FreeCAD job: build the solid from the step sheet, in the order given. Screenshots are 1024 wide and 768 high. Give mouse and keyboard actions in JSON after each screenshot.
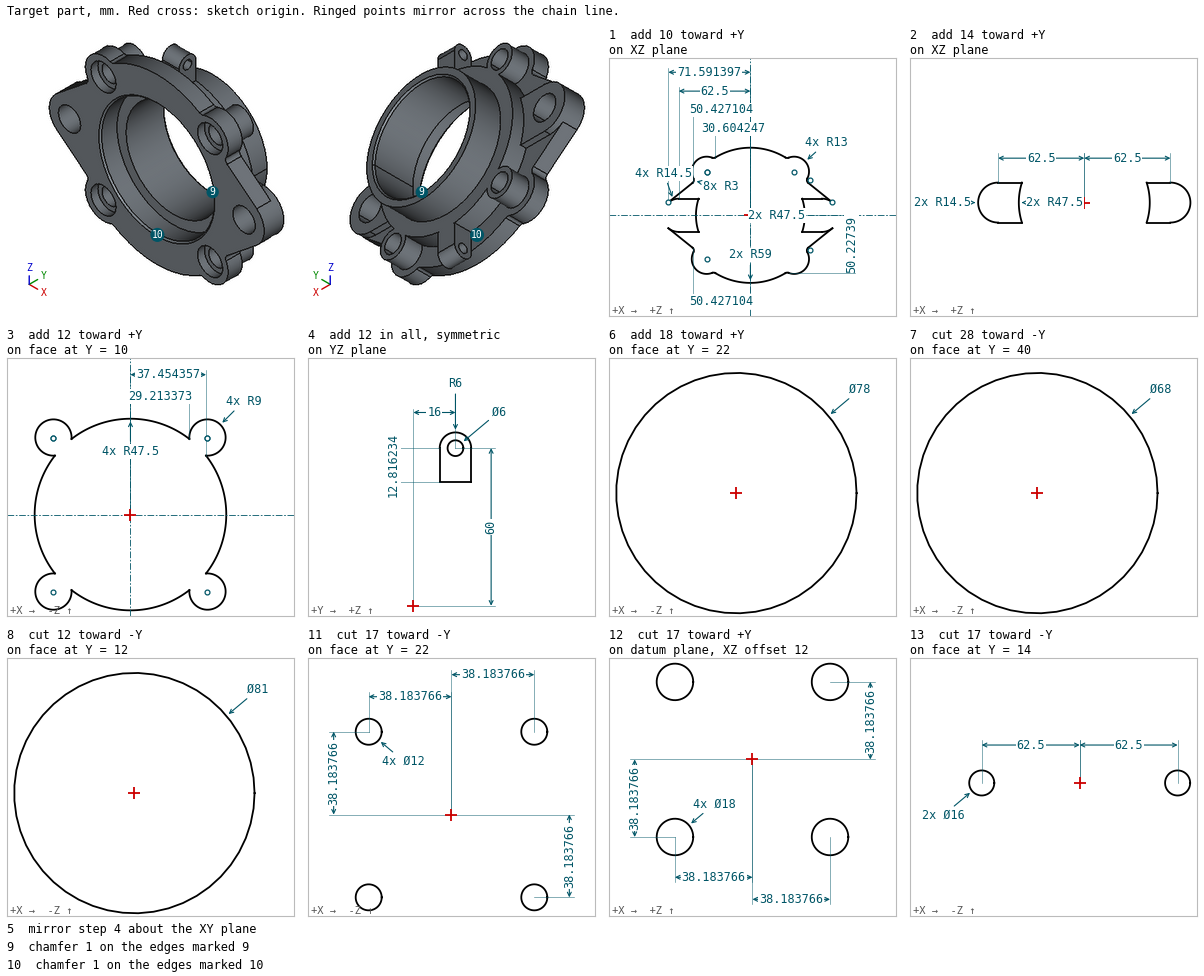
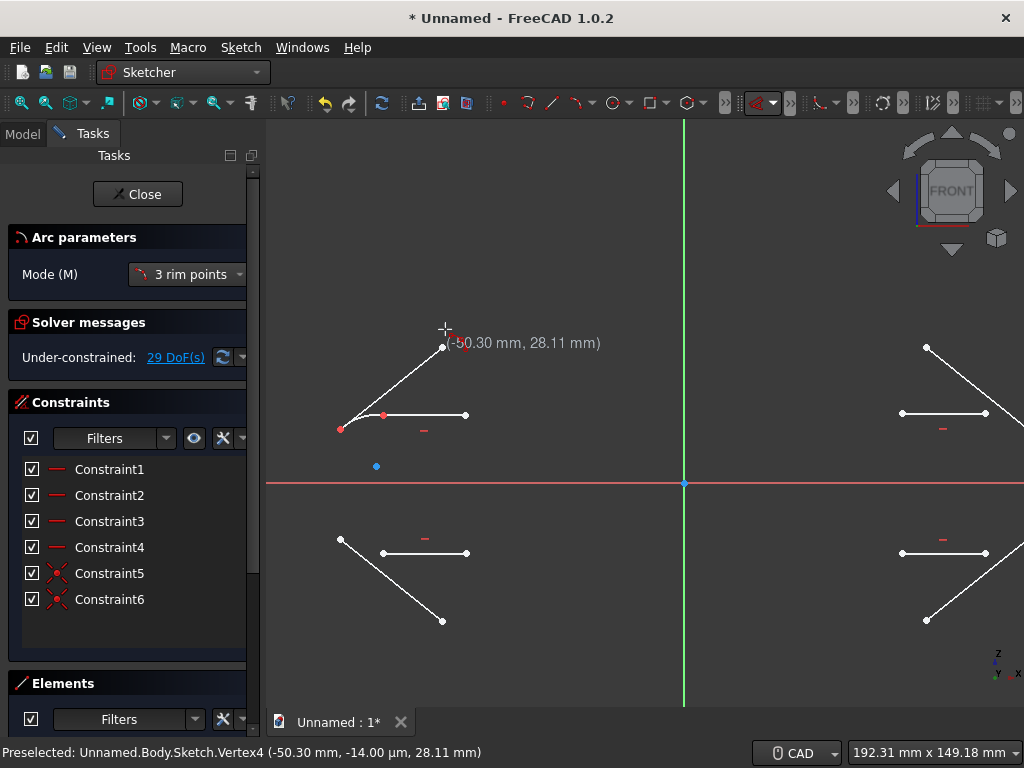
{"action": "left_click", "coordinate": [445, 329]}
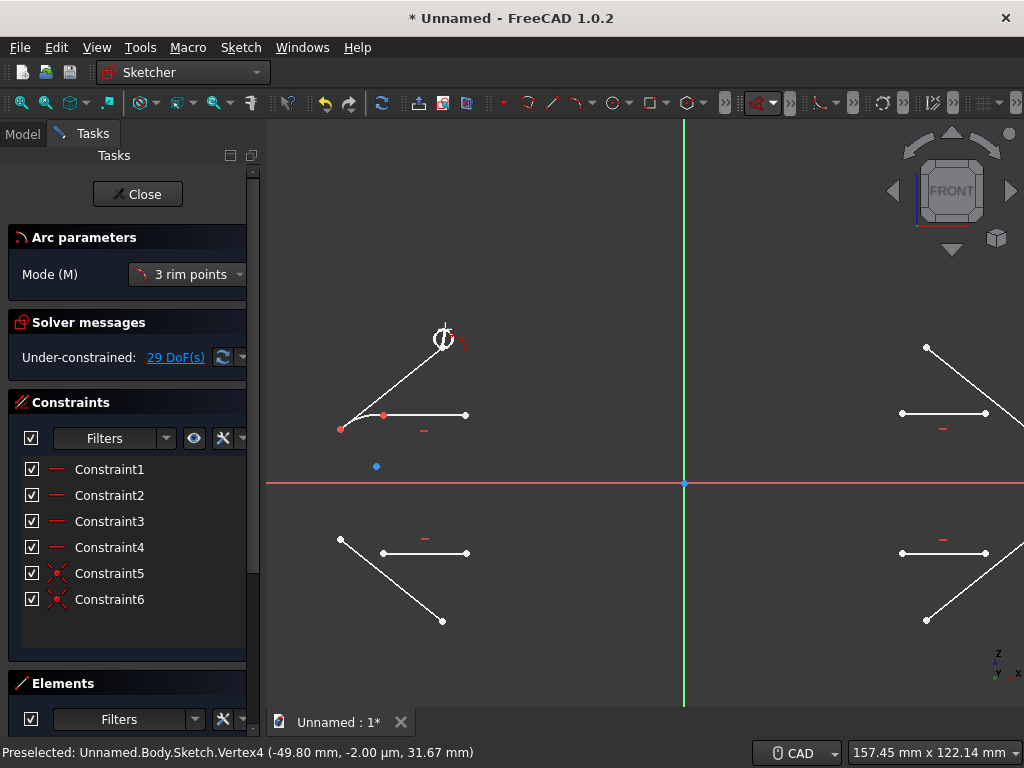
{"action": "scroll", "coordinate": [447, 339], "scroll_direction": "up", "scroll_amount": 8}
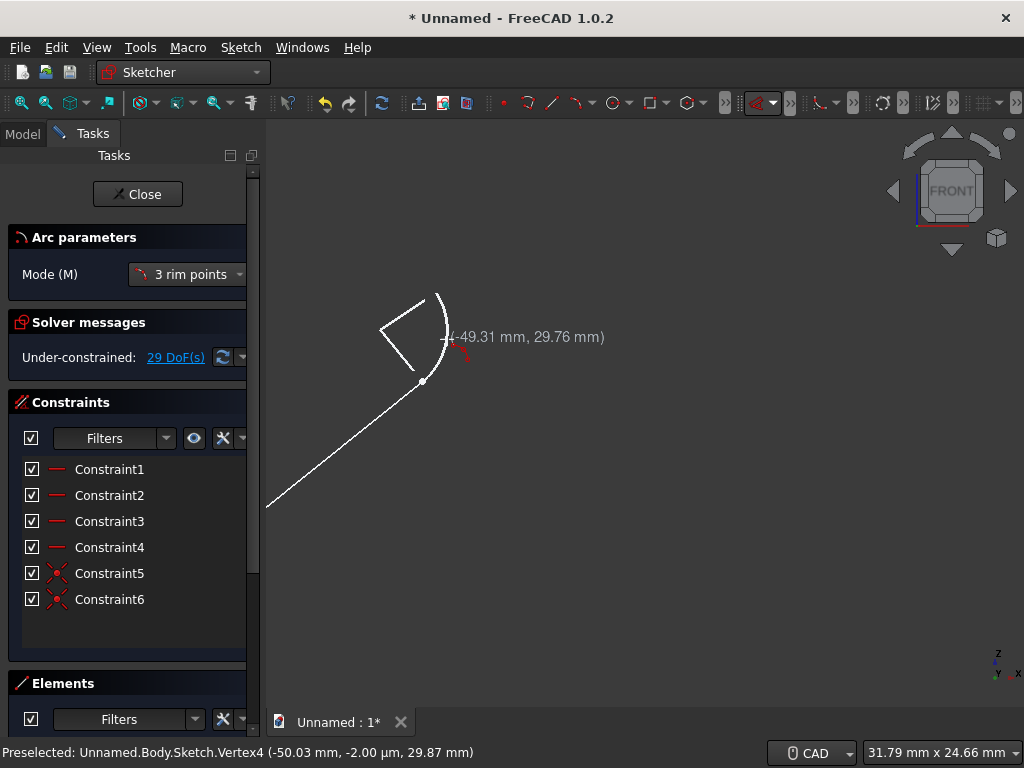
{"action": "left_click", "coordinate": [445, 335]}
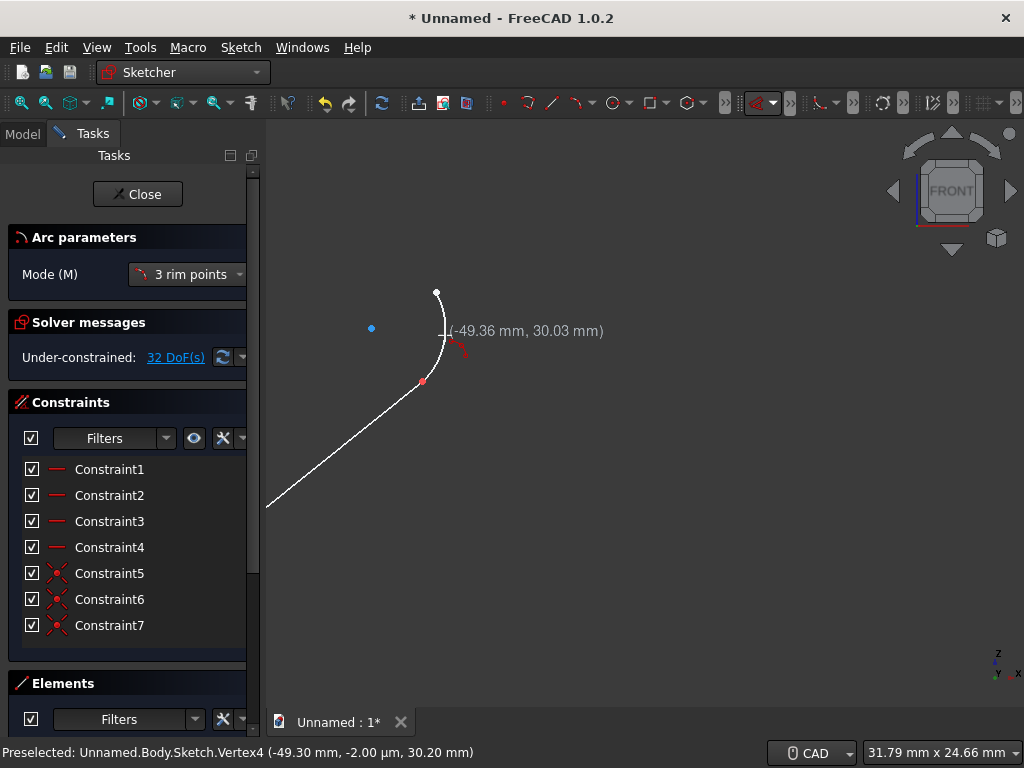
{"action": "scroll", "coordinate": [446, 333], "scroll_direction": "down", "scroll_amount": 11}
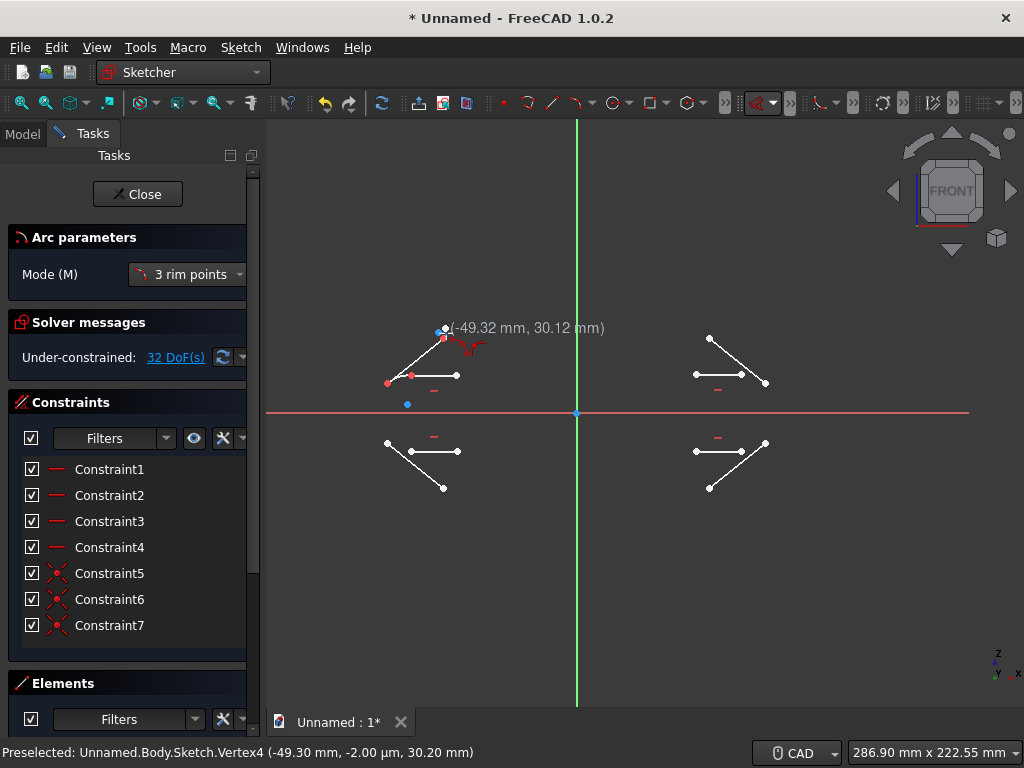
{"action": "scroll", "coordinate": [445, 328], "scroll_direction": "up", "scroll_amount": 4}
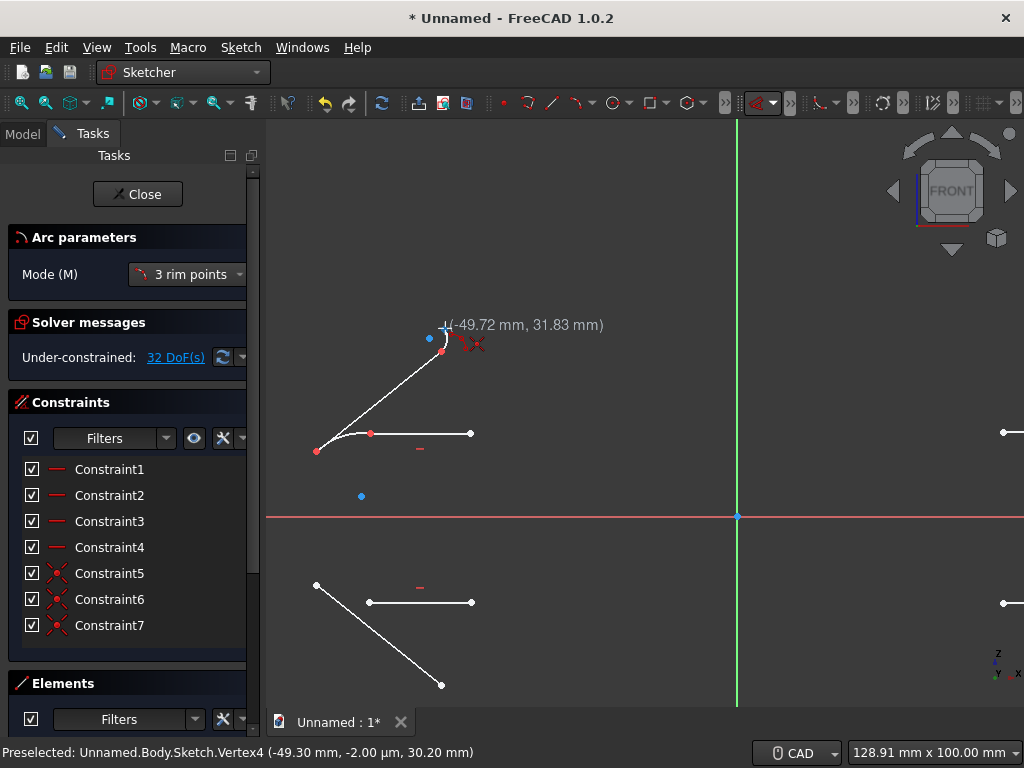
{"action": "left_click", "coordinate": [445, 330]}
{"action": "left_click", "coordinate": [542, 221]}
{"action": "left_click", "coordinate": [456, 241]}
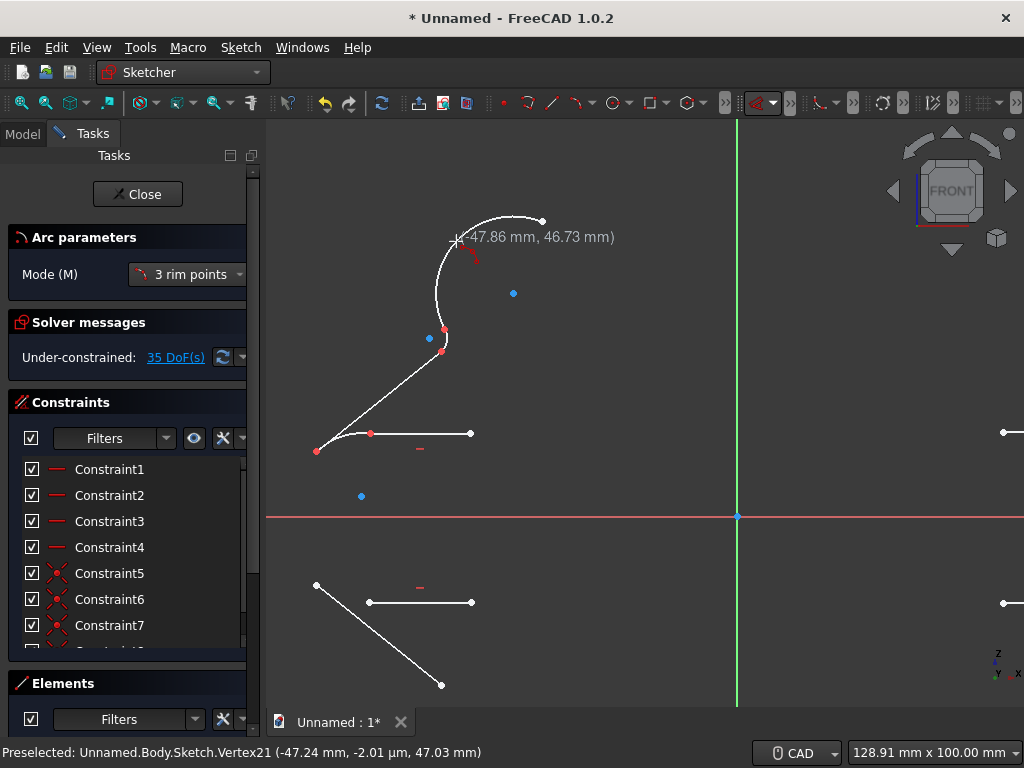
{"action": "left_click", "coordinate": [542, 222]}
{"action": "left_click", "coordinate": [557, 220]}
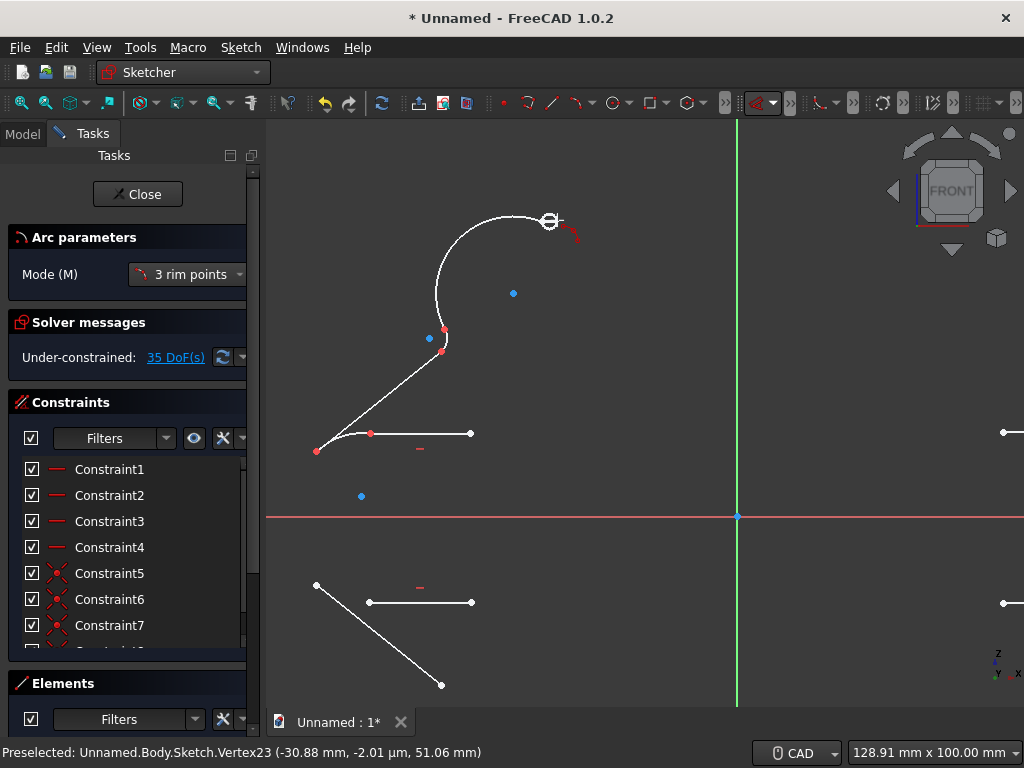
{"action": "scroll", "coordinate": [550, 223], "scroll_direction": "up", "scroll_amount": 11}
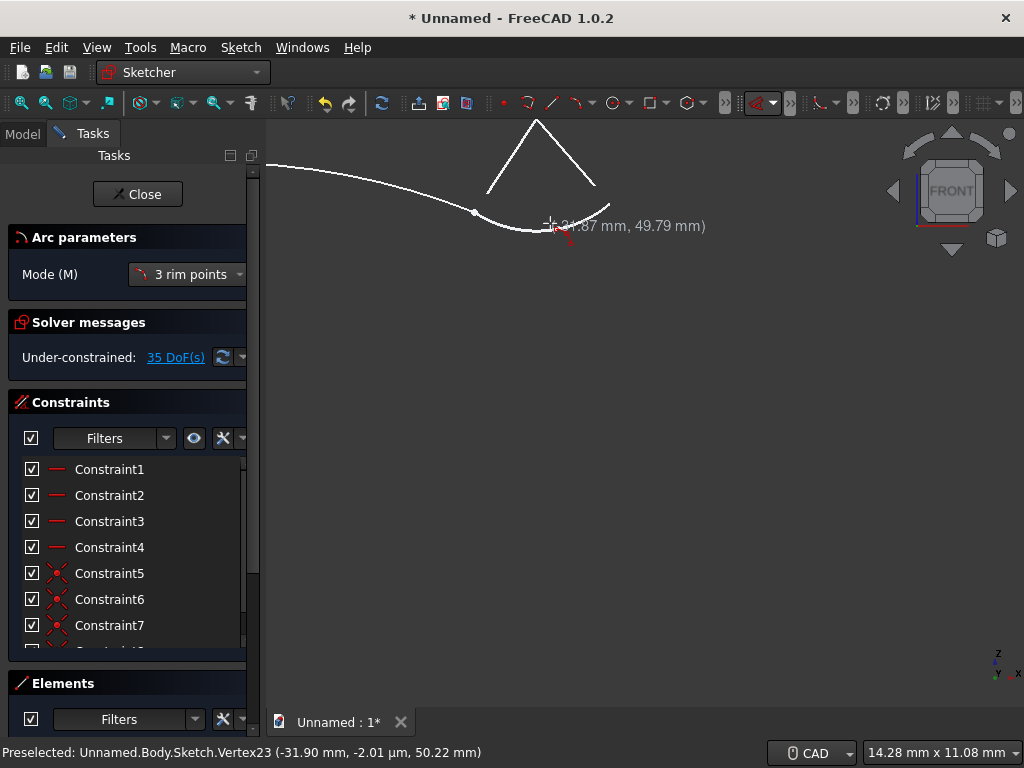
{"action": "left_click", "coordinate": [544, 219]}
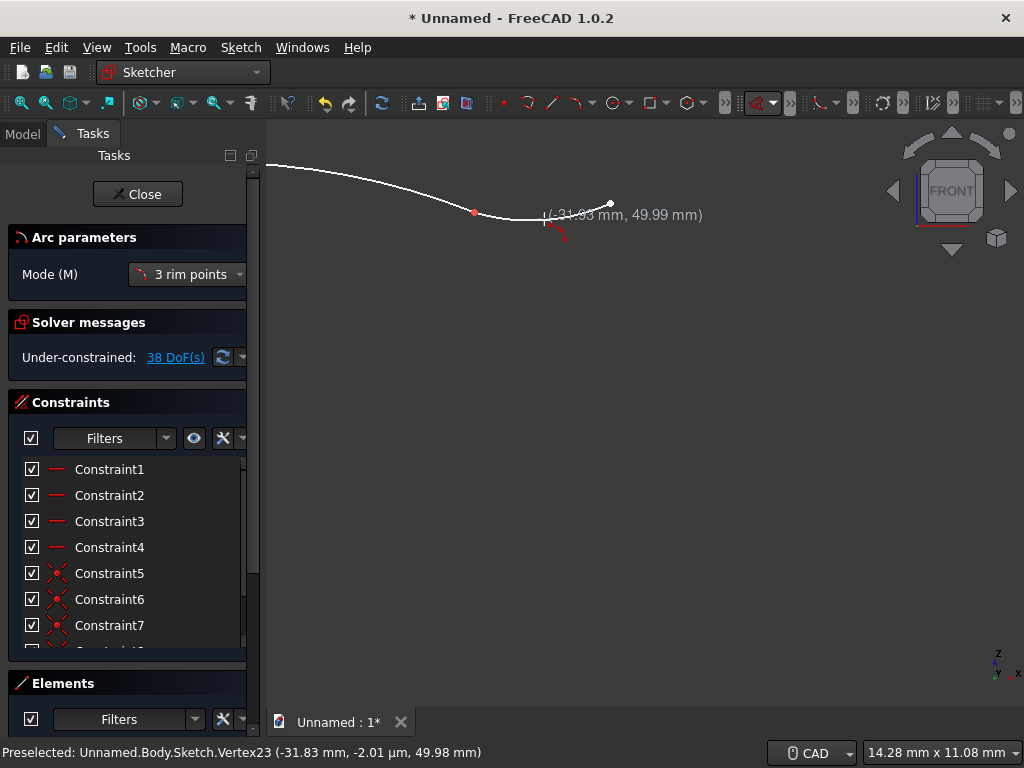
{"action": "scroll", "coordinate": [489, 284], "scroll_direction": "down", "scroll_amount": 15}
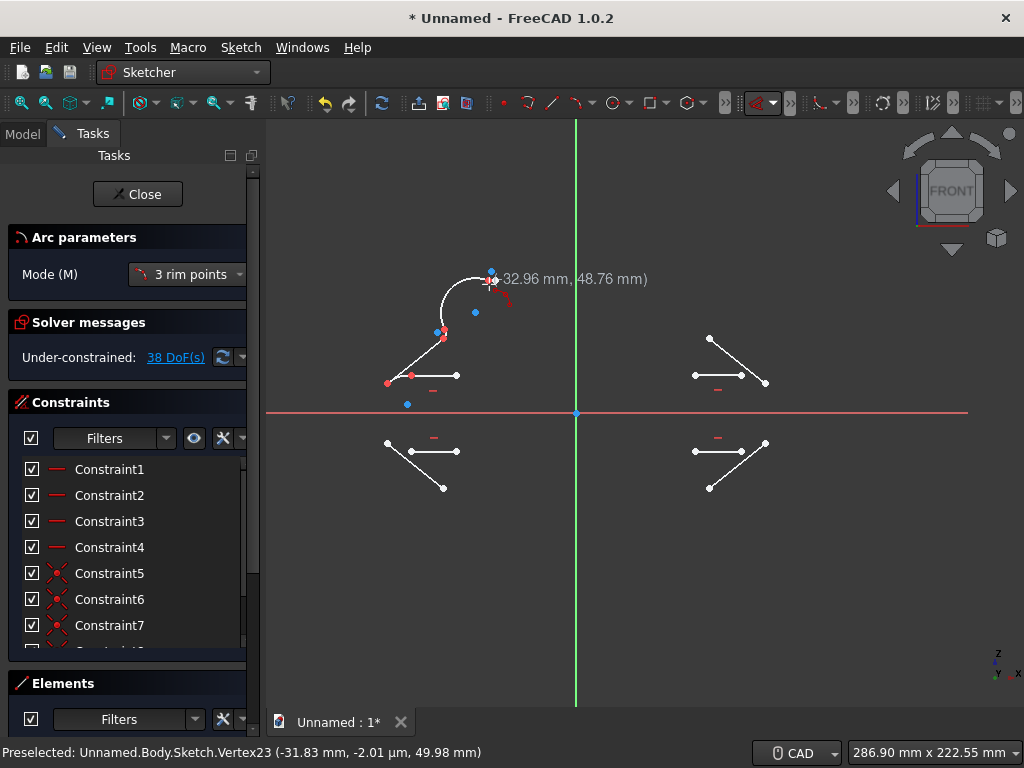
{"action": "scroll", "coordinate": [496, 280], "scroll_direction": "up", "scroll_amount": 5}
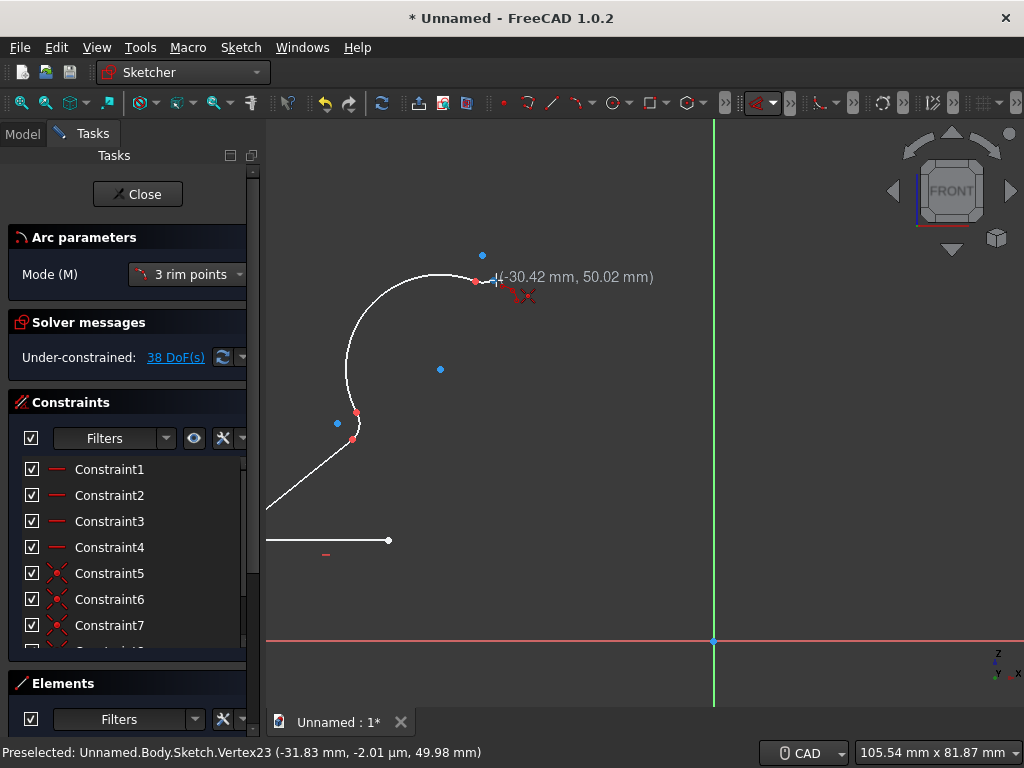
{"action": "left_click", "coordinate": [494, 280]}